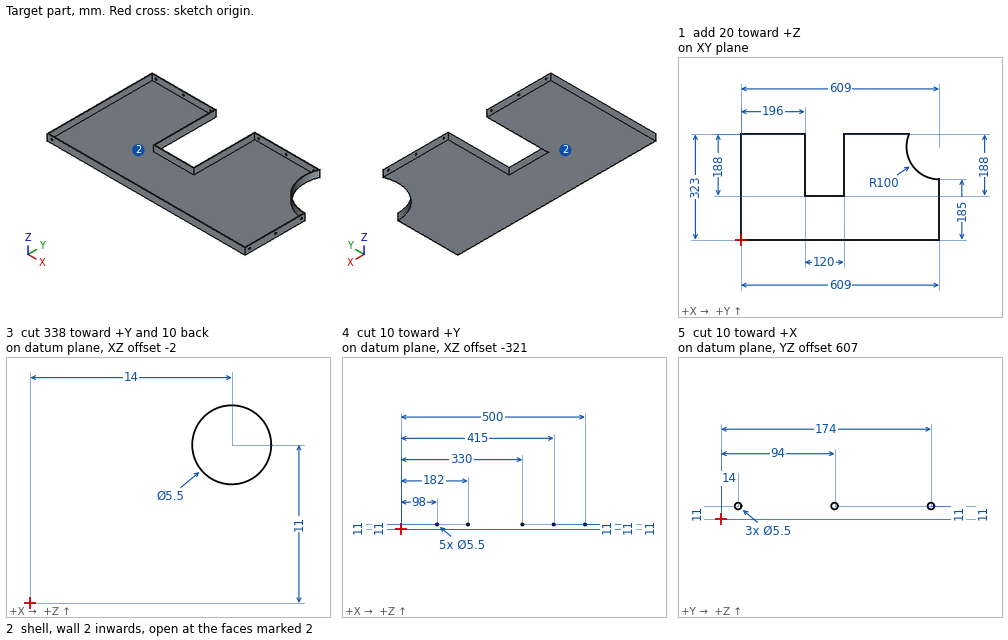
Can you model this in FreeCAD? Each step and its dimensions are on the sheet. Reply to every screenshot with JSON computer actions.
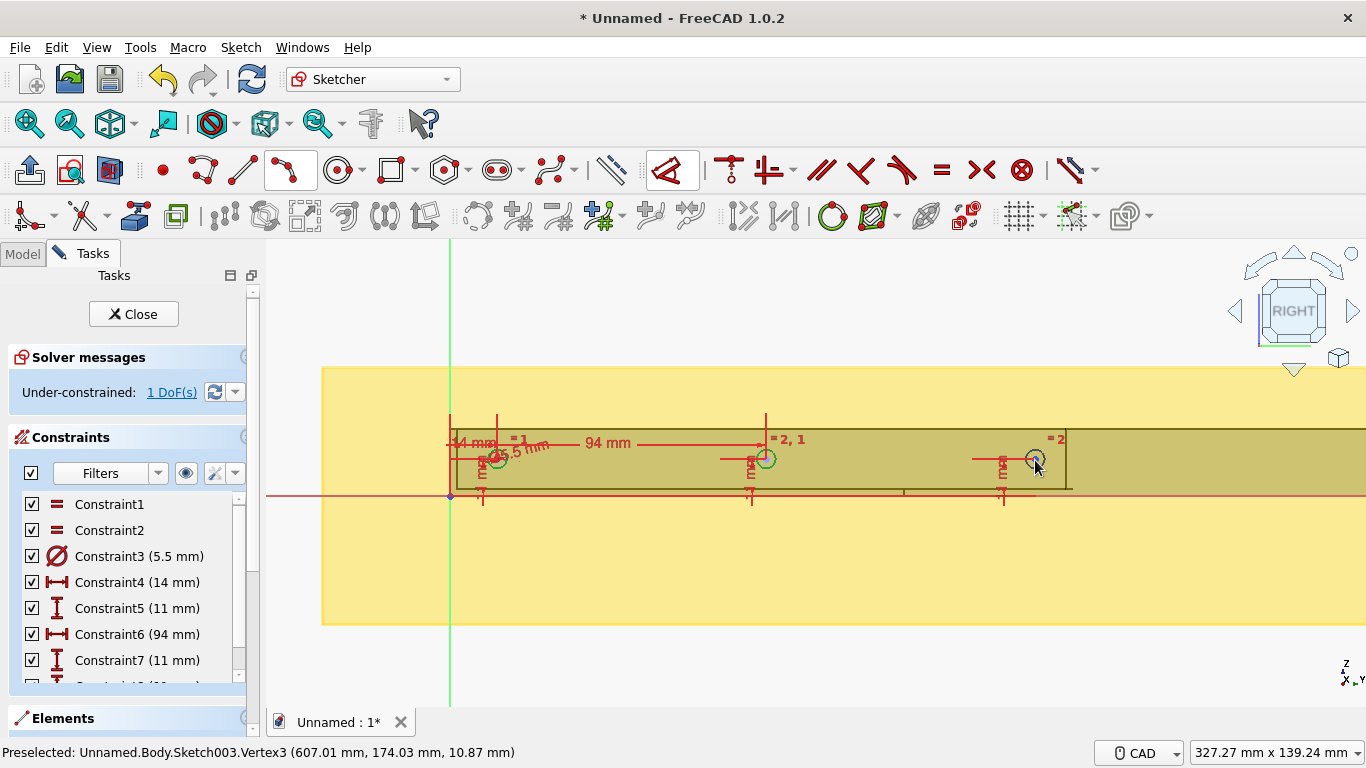
{"action": "left_click", "coordinate": [1035, 459]}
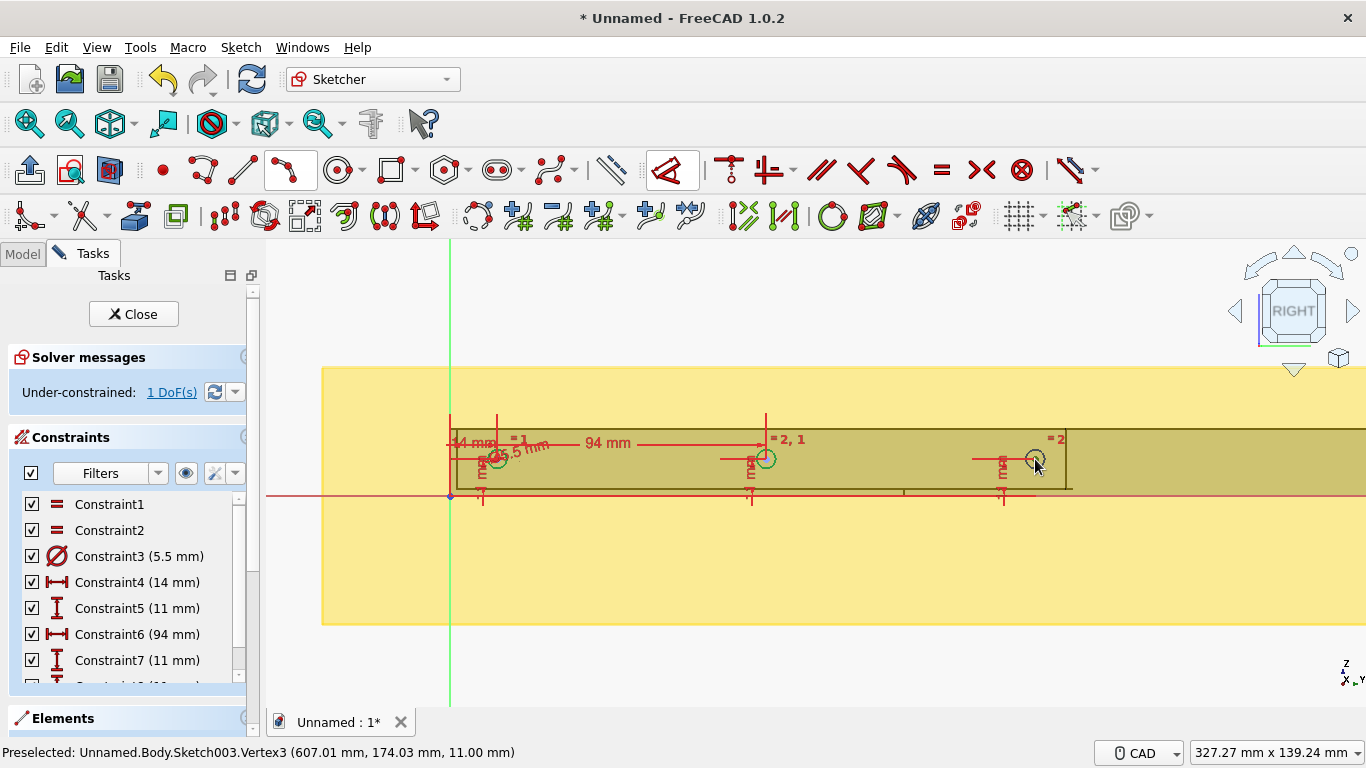
{"action": "key", "text": "l"}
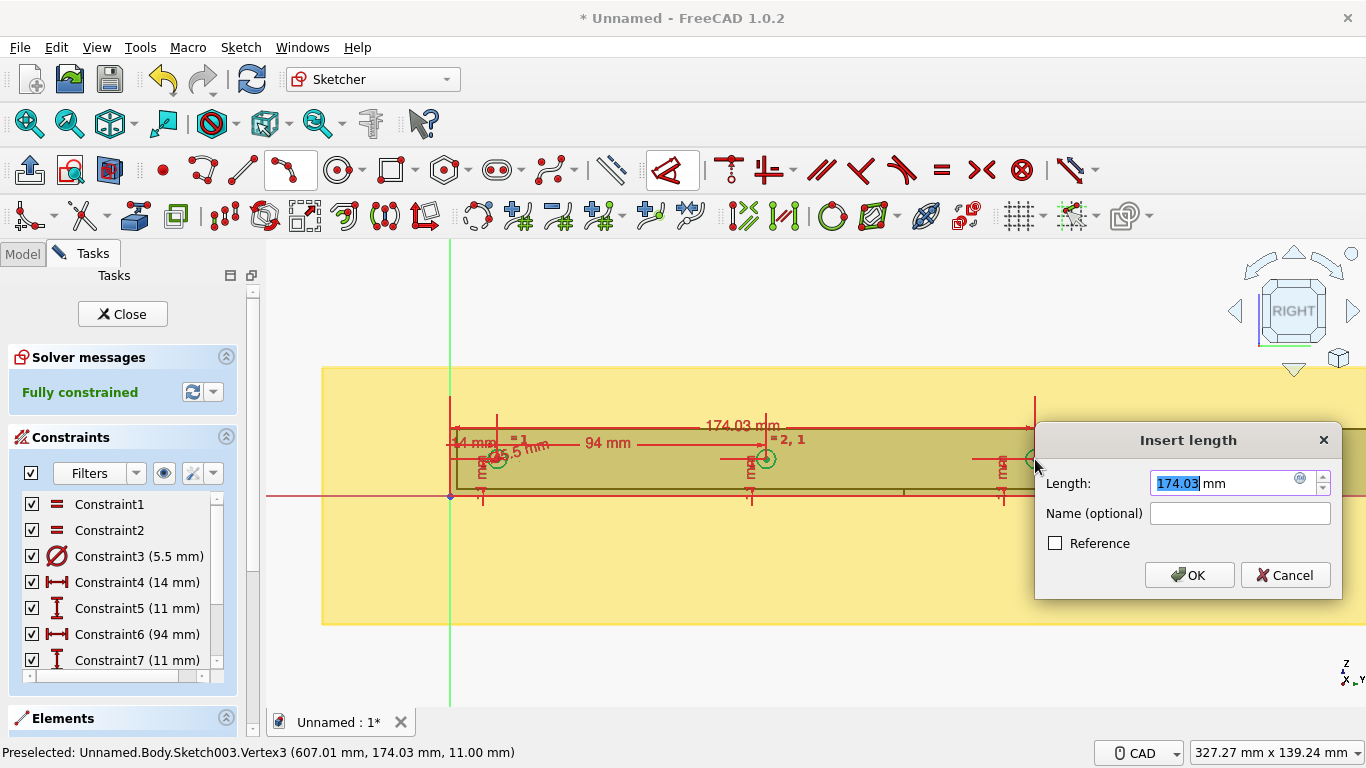
{"action": "type", "text": "174"}
{"action": "key", "text": "Return"}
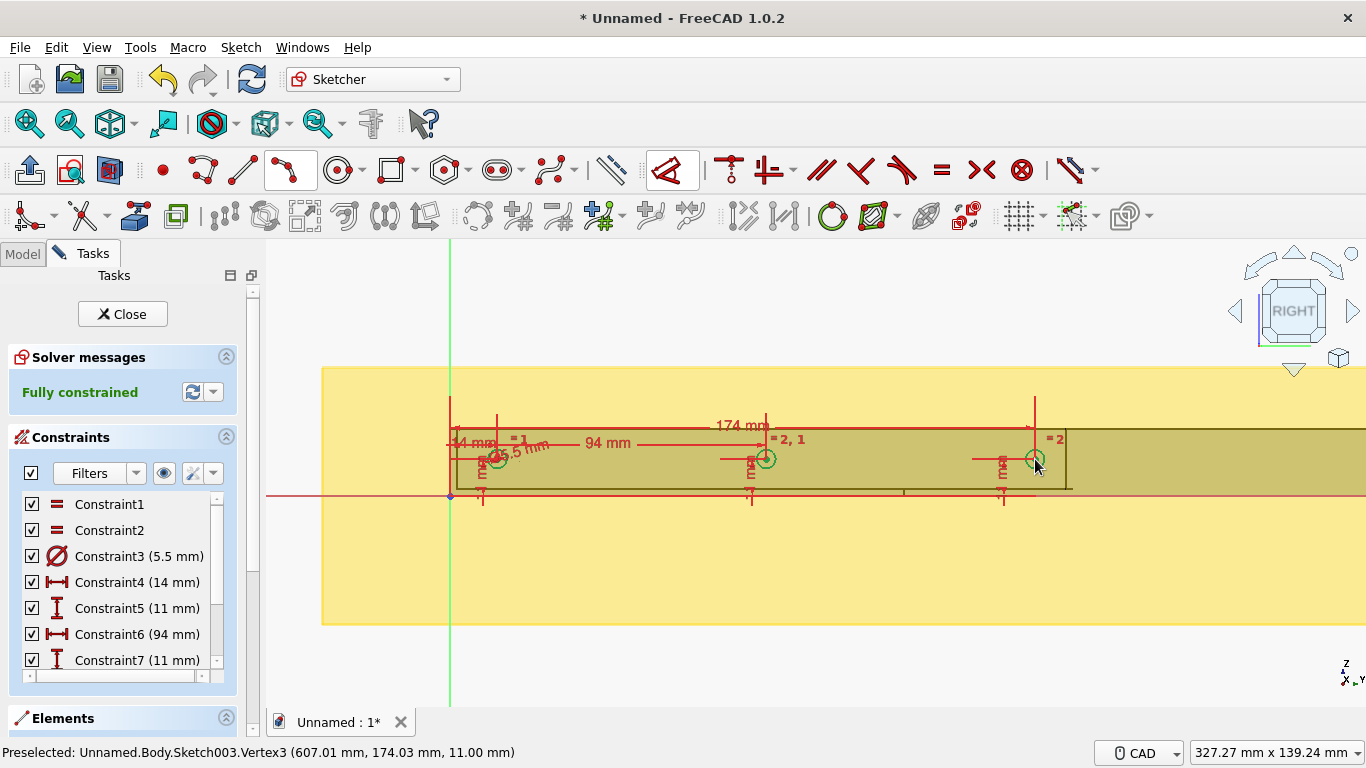
{"action": "left_click", "coordinate": [123, 314]}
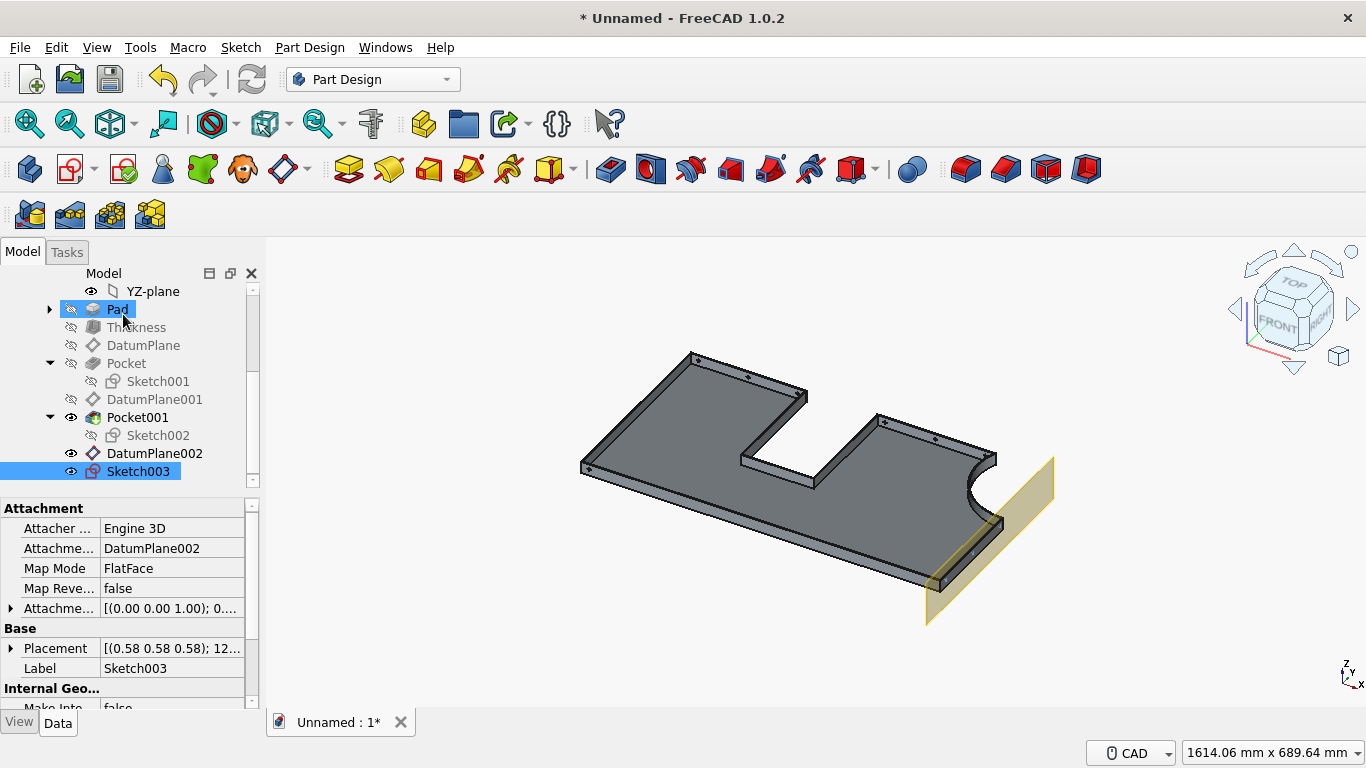
{"action": "left_click", "coordinate": [612, 170]}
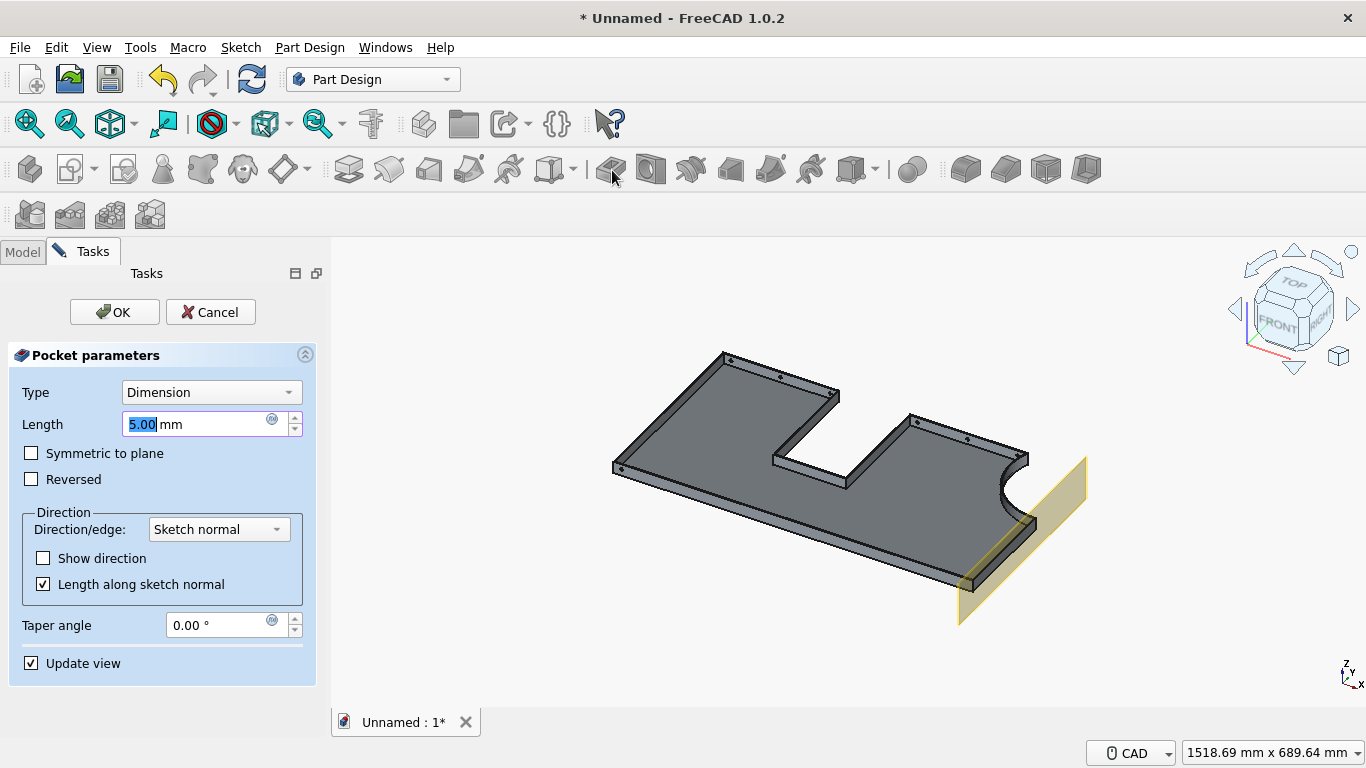
{"action": "type", "text": "10"}
{"action": "key", "text": "Tab"}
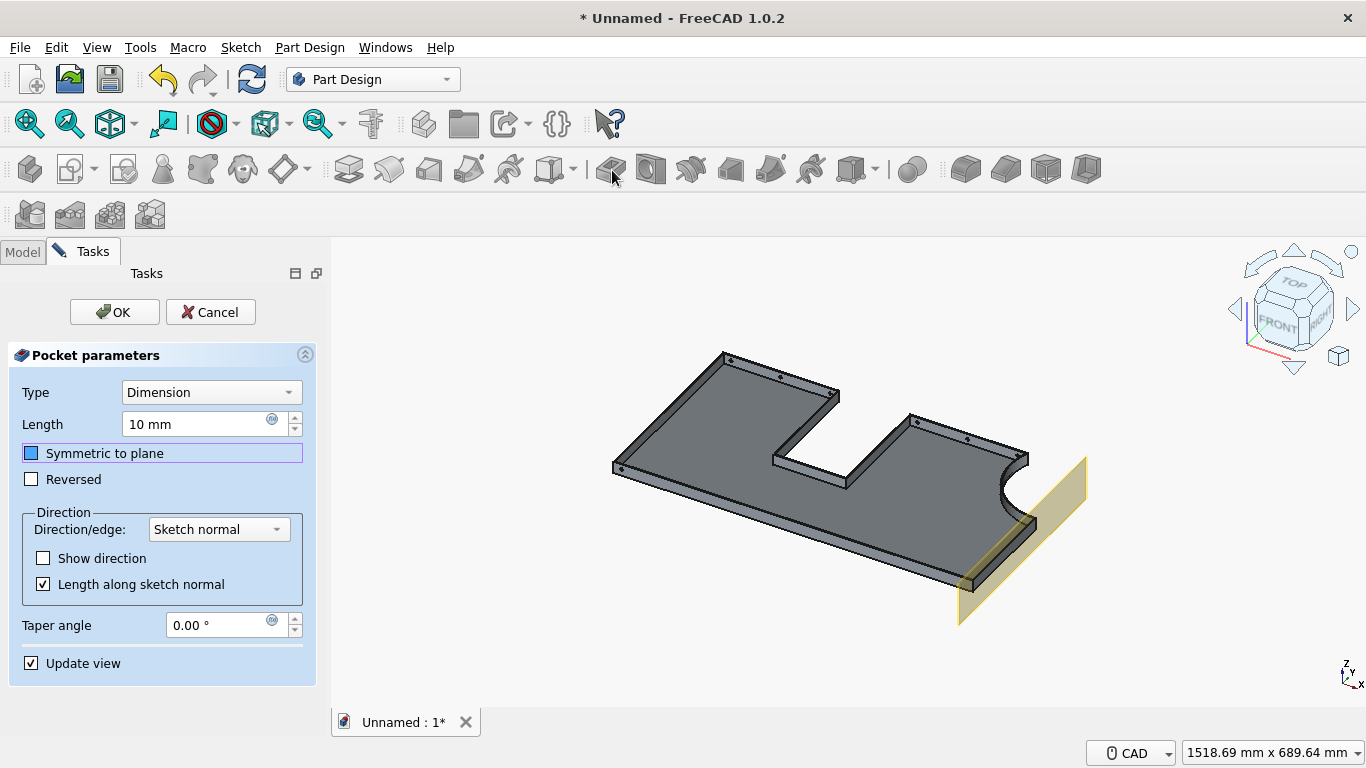
{"action": "left_click", "coordinate": [30, 479]}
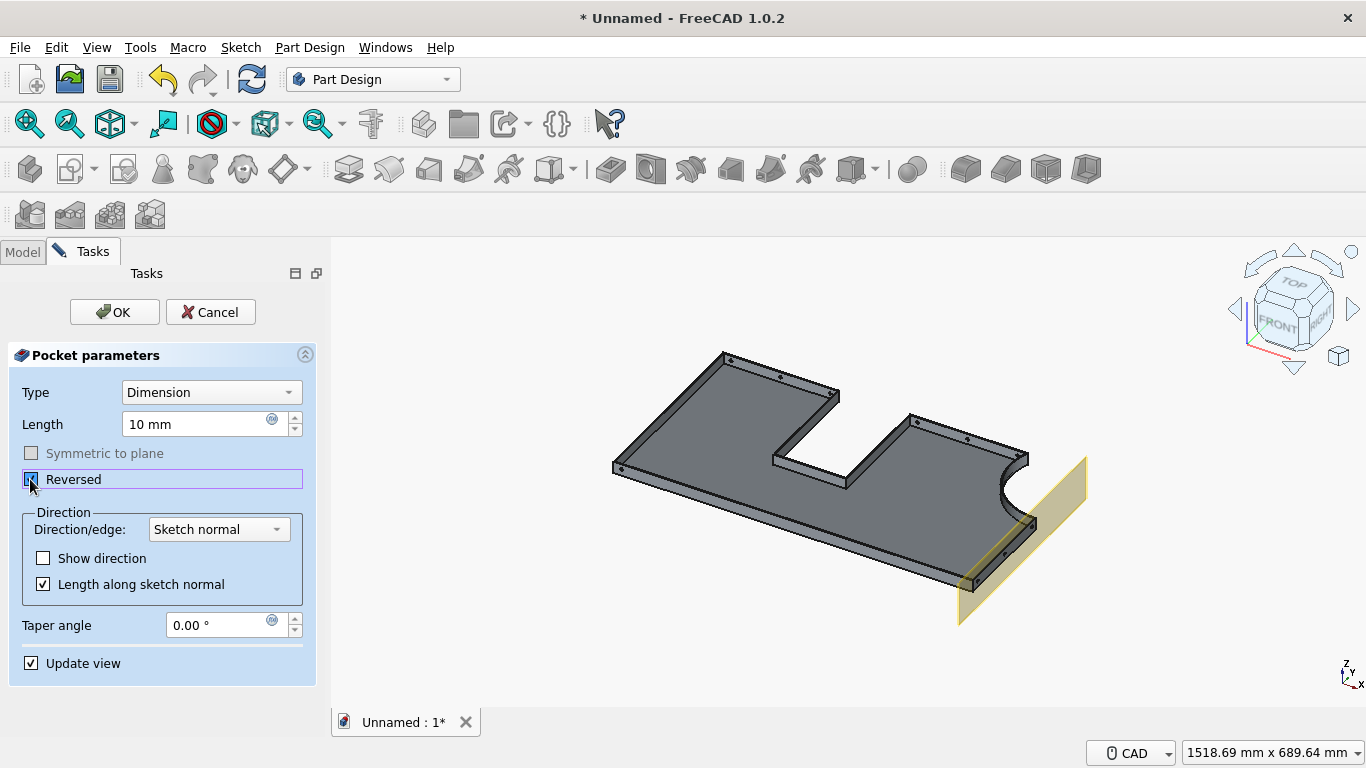
{"action": "left_click", "coordinate": [115, 312]}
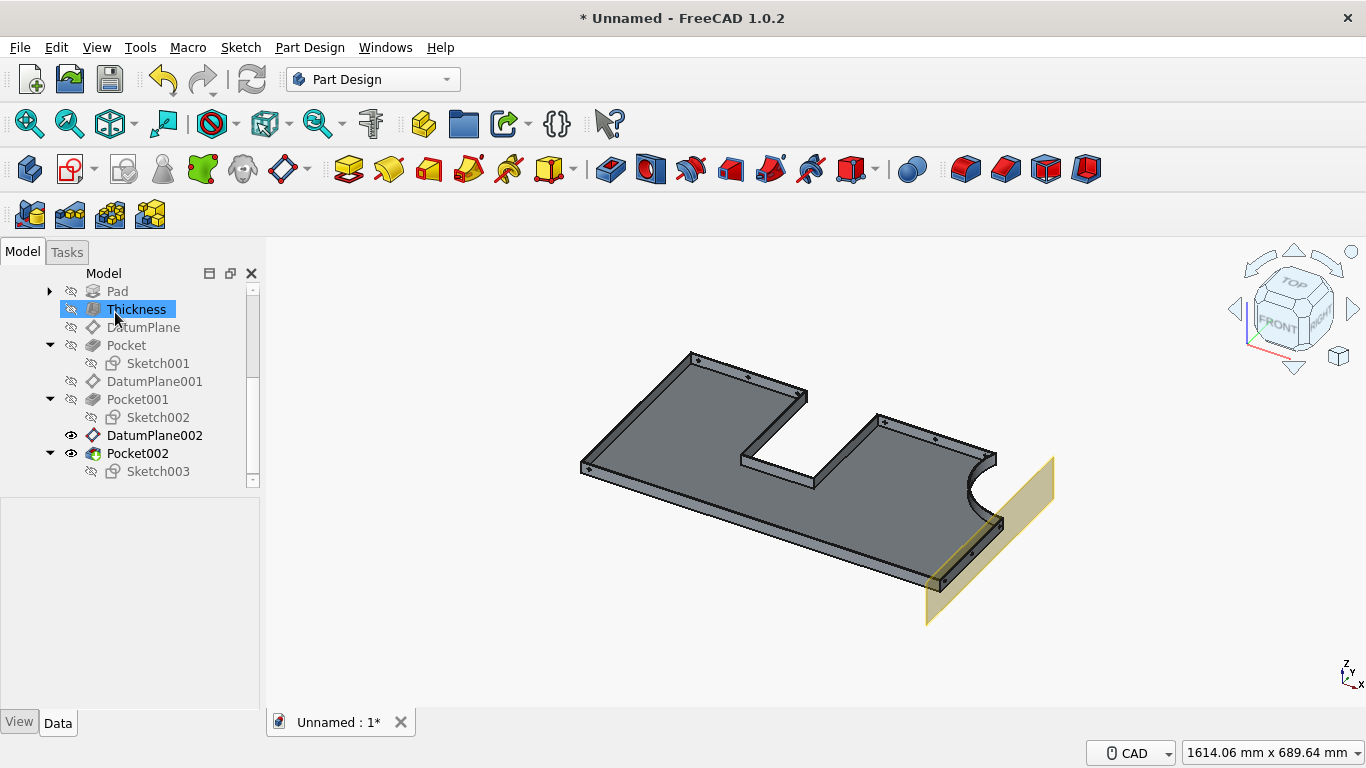
{"action": "left_click", "coordinate": [116, 435]}
{"action": "key", "text": "space"}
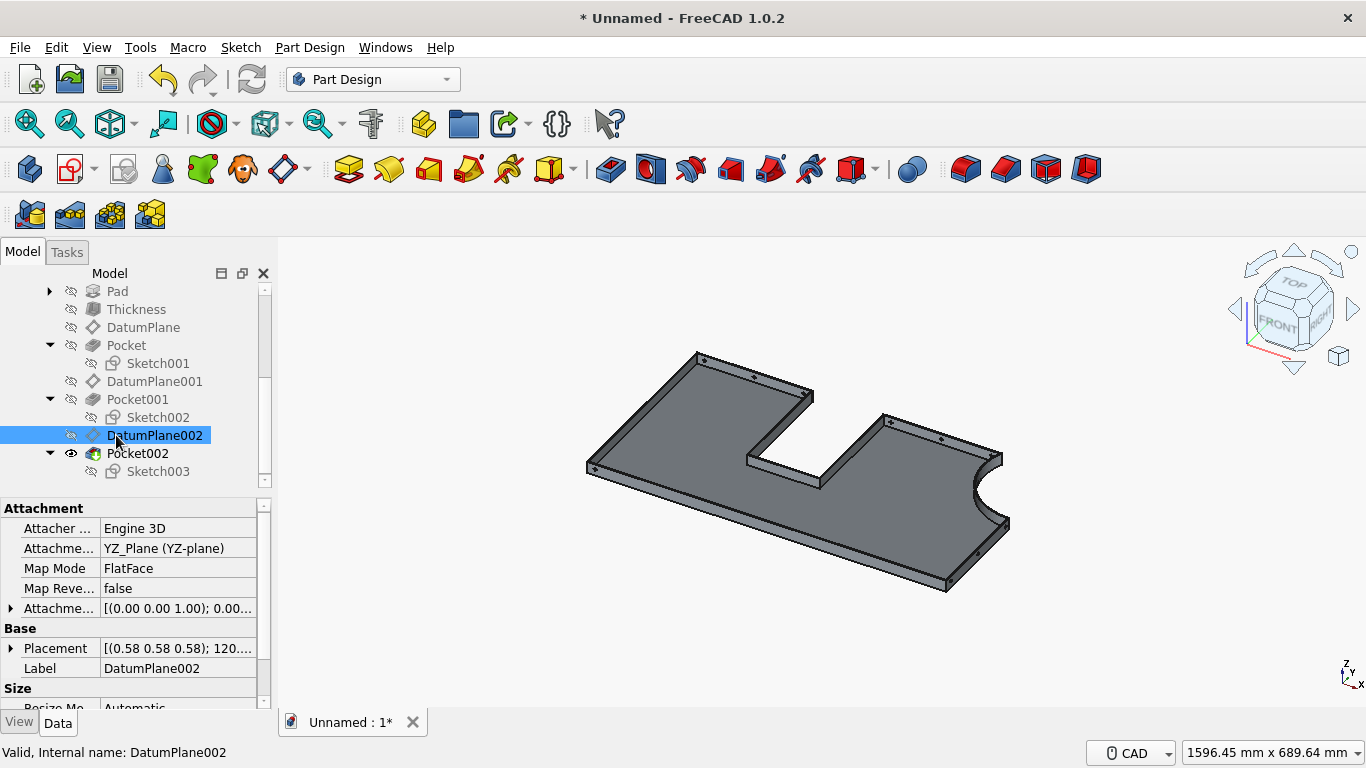
{"action": "key", "text": "0"}